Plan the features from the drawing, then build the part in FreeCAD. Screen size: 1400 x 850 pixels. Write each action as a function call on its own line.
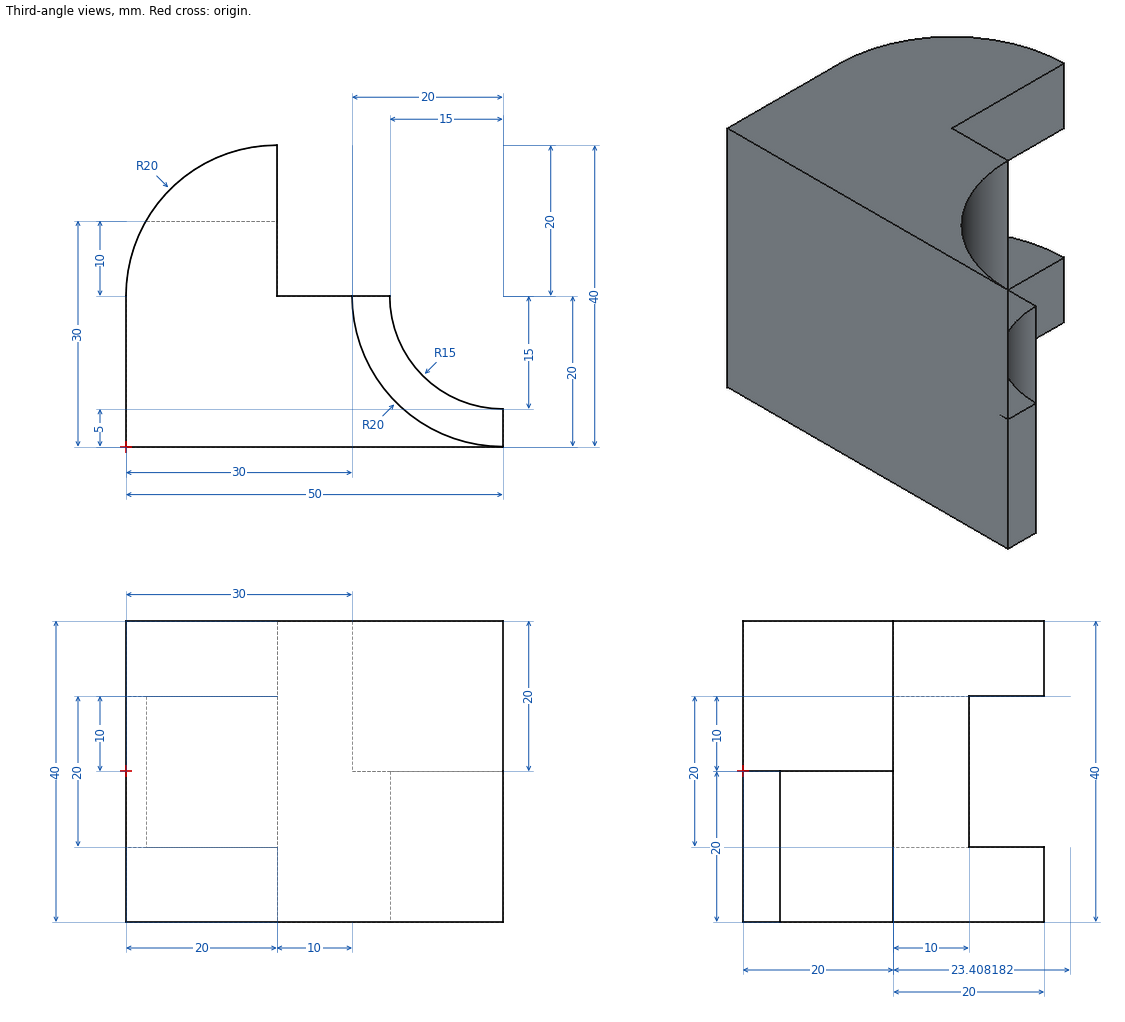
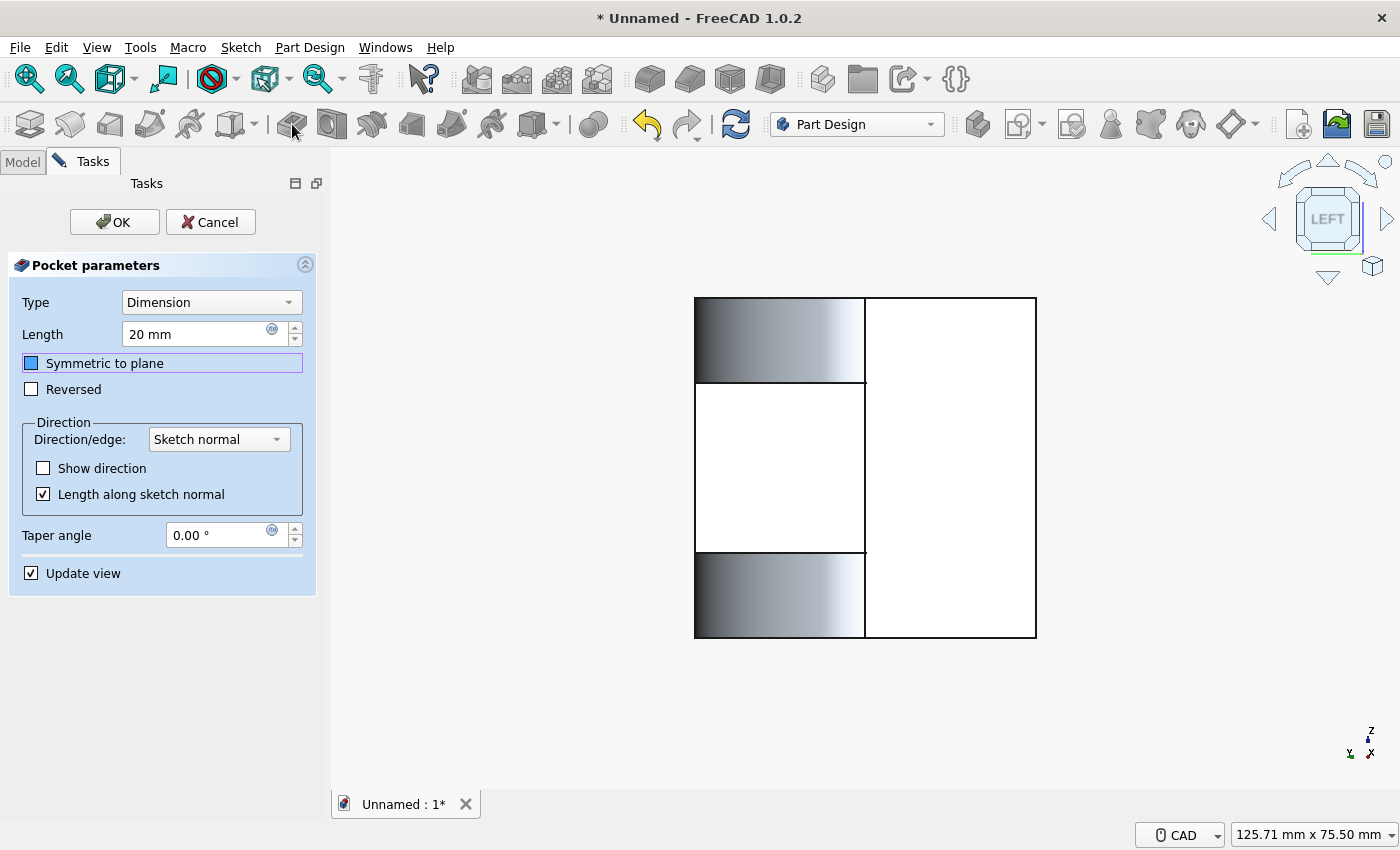
click(115, 222)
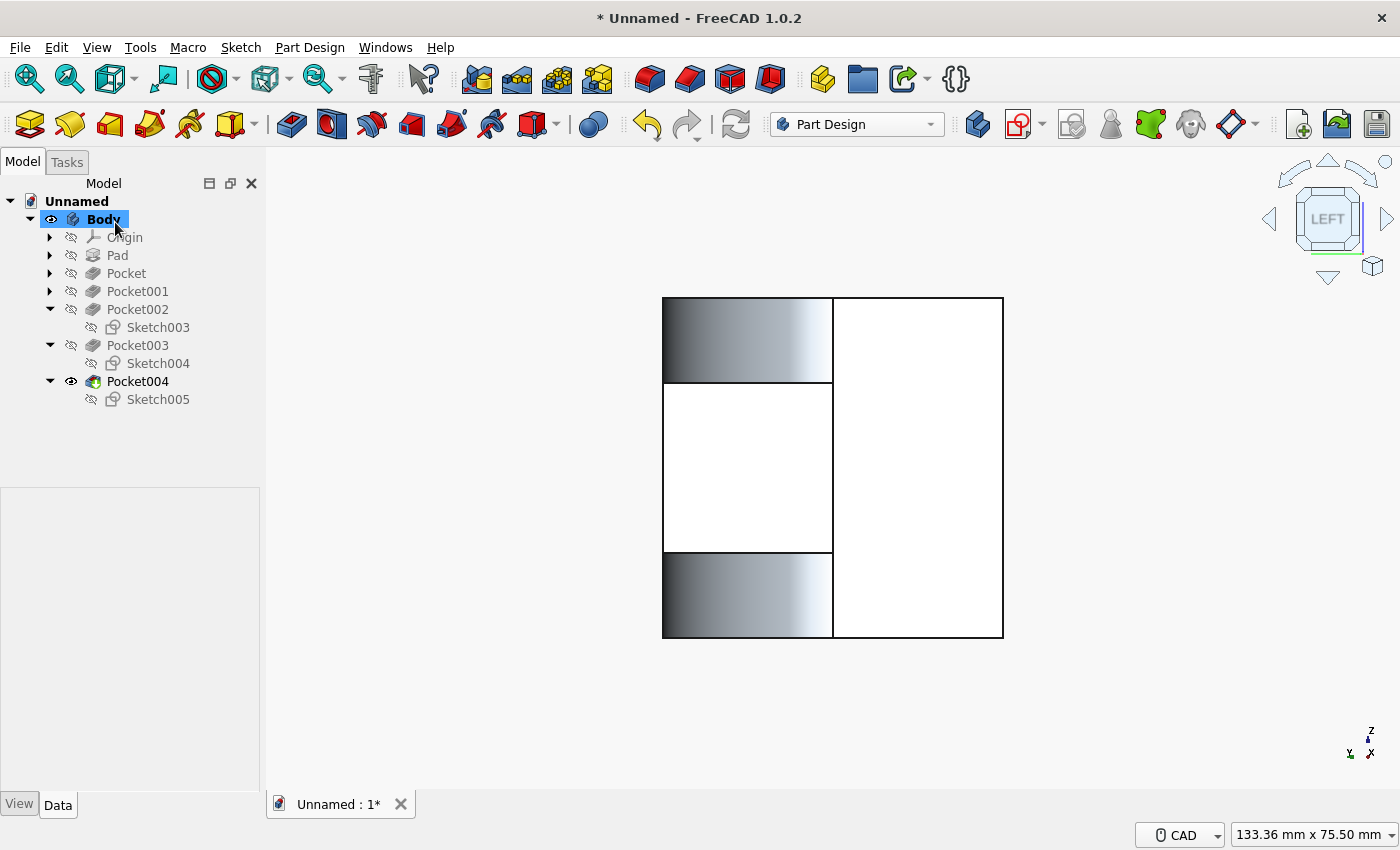
key(4)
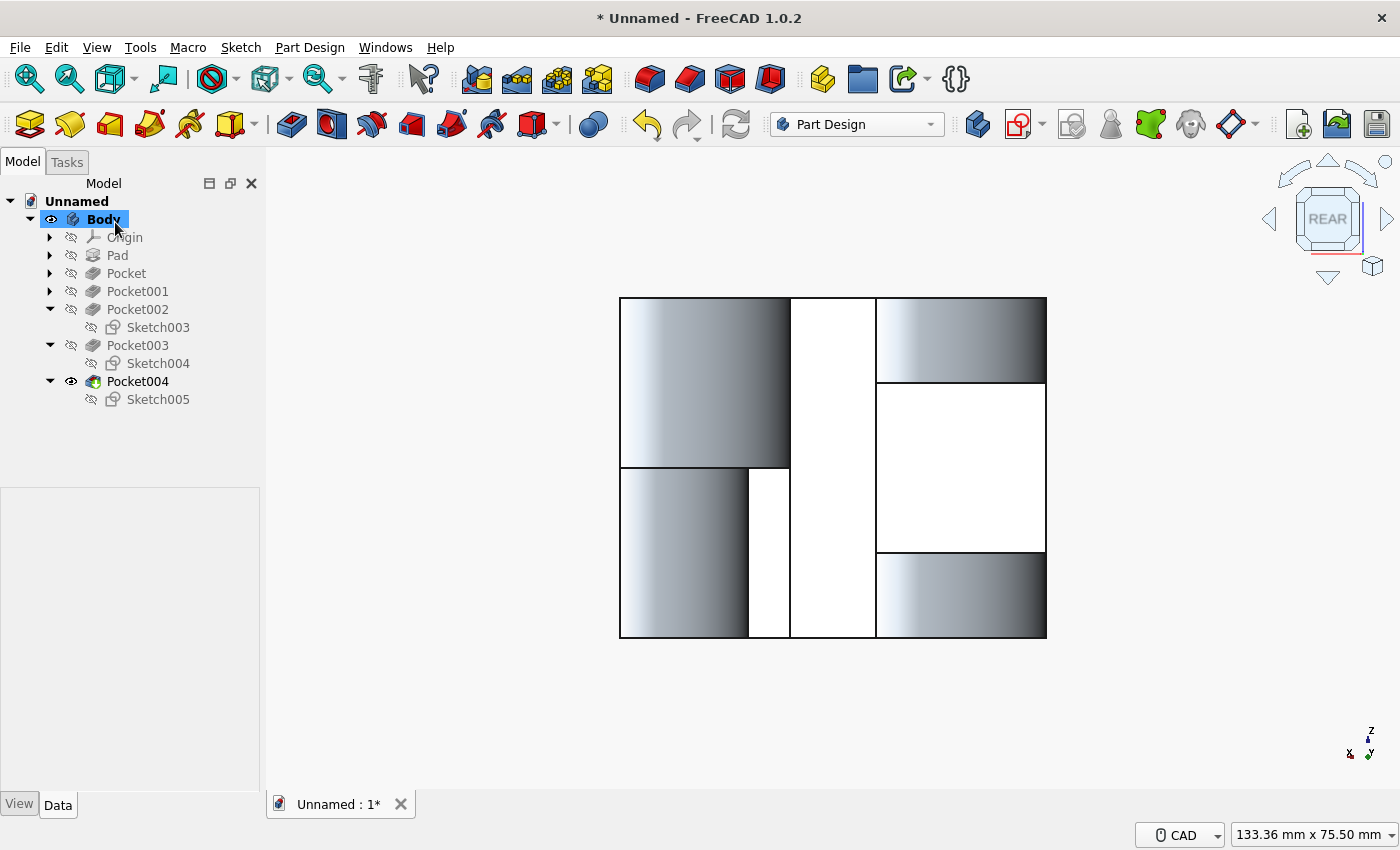
click(833, 370)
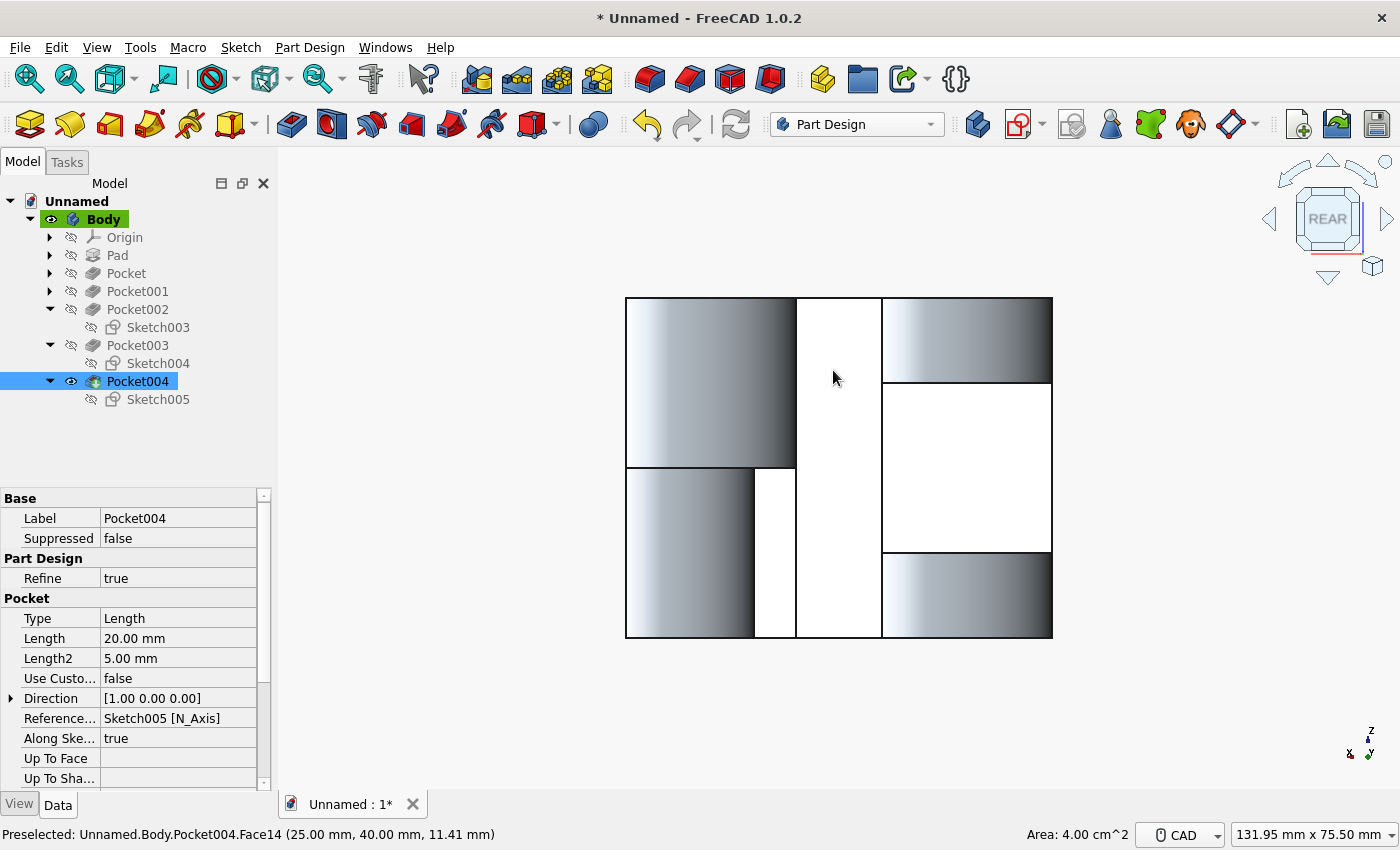
click(1018, 124)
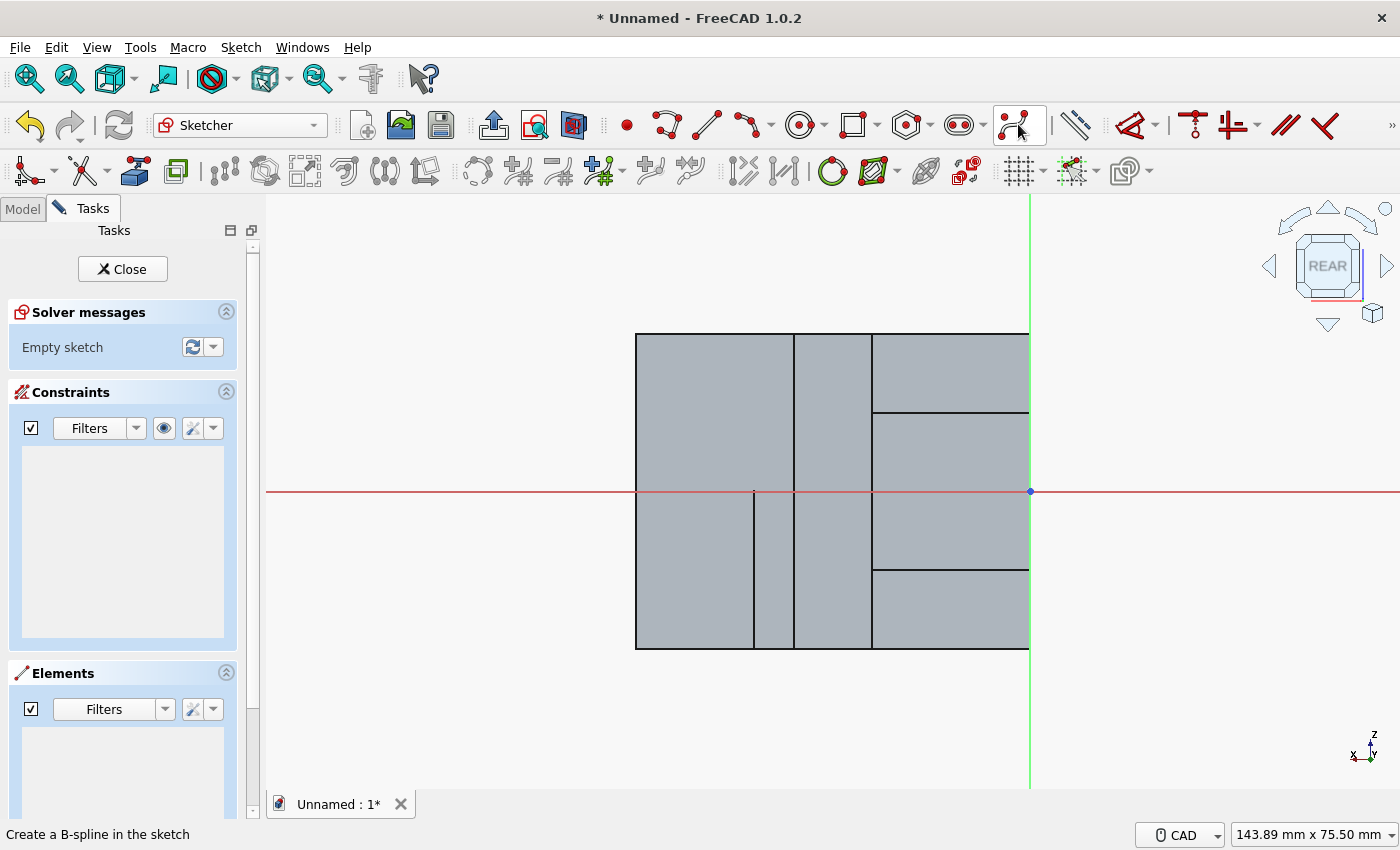
key(g)
key(r)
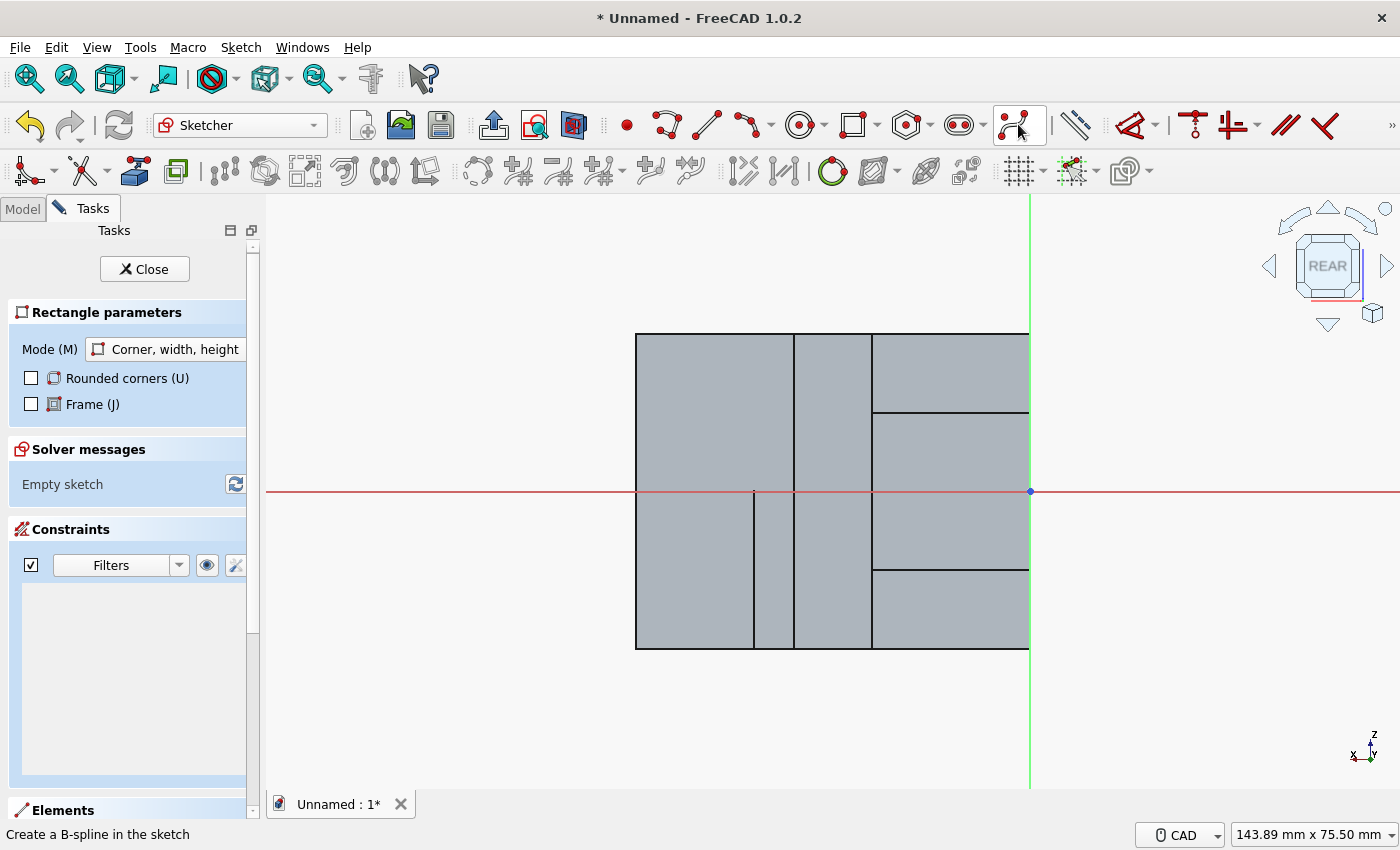
click(794, 334)
move(872, 649)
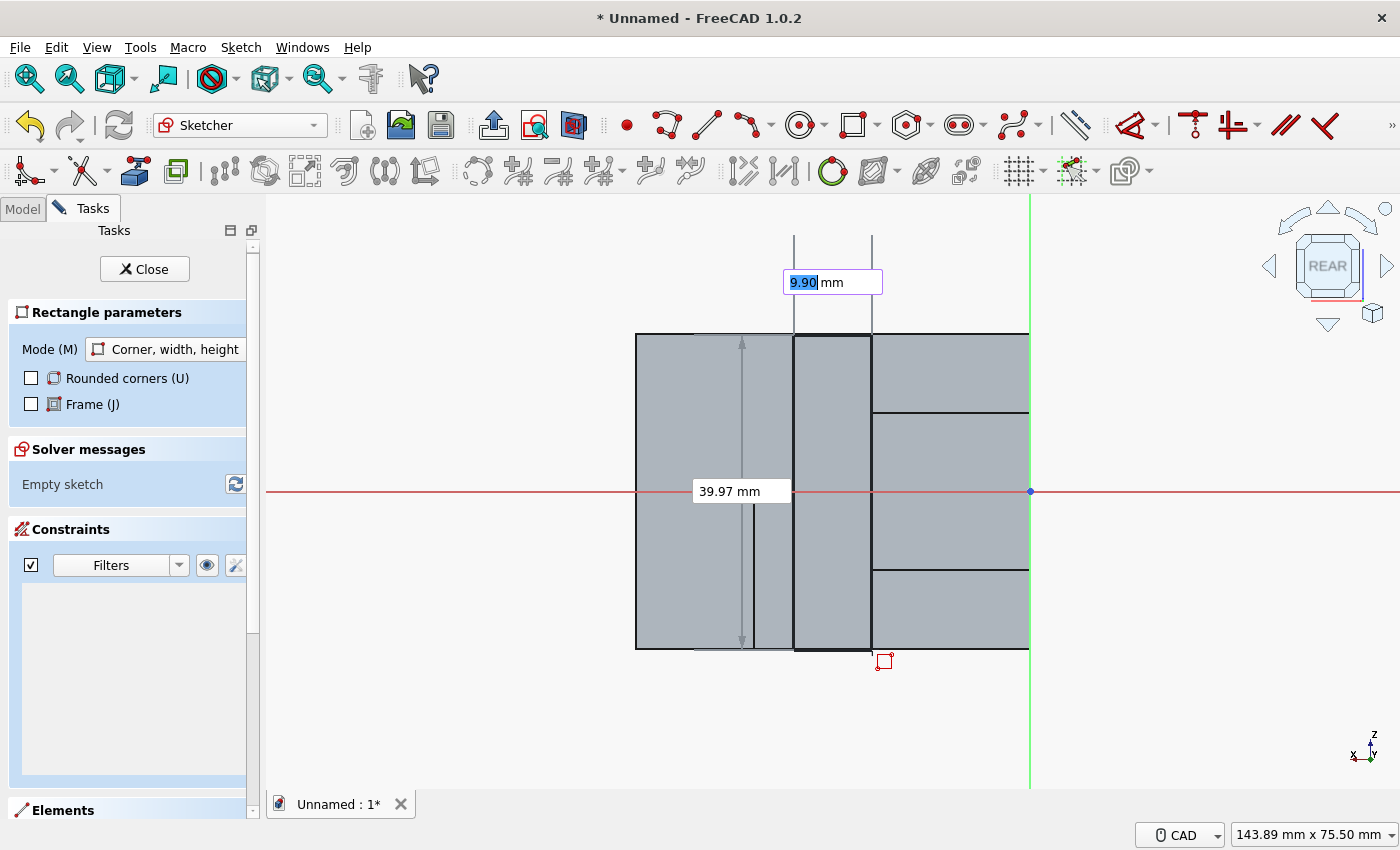
text(10)
key(Tab)
text(40)
key(Return)
key(Escape)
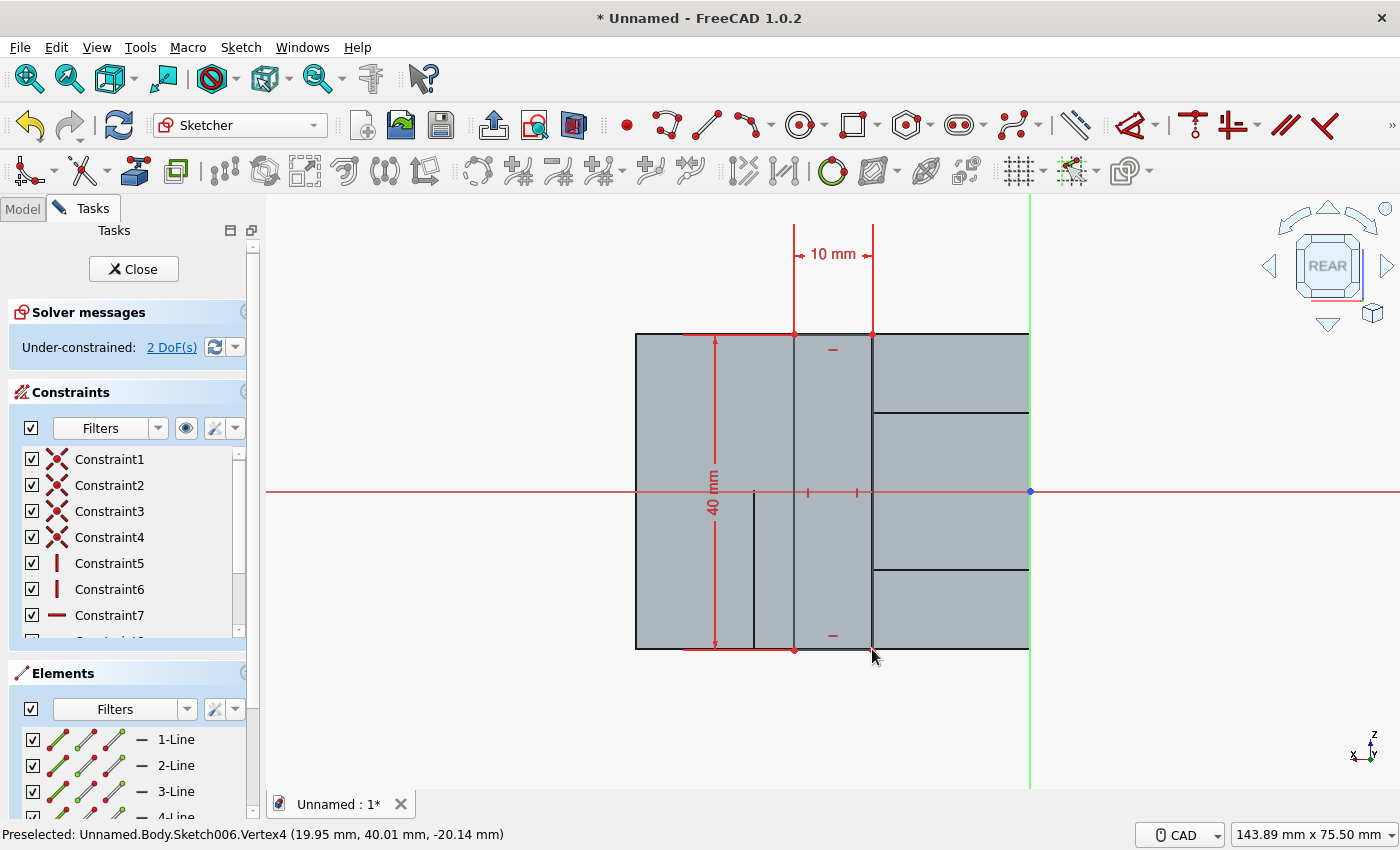
click(1130, 126)